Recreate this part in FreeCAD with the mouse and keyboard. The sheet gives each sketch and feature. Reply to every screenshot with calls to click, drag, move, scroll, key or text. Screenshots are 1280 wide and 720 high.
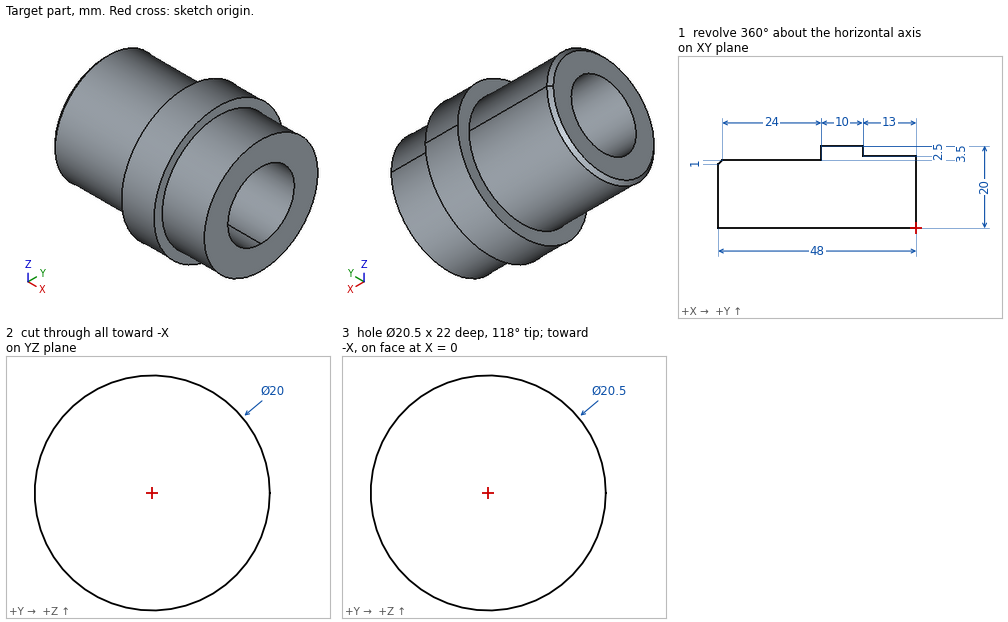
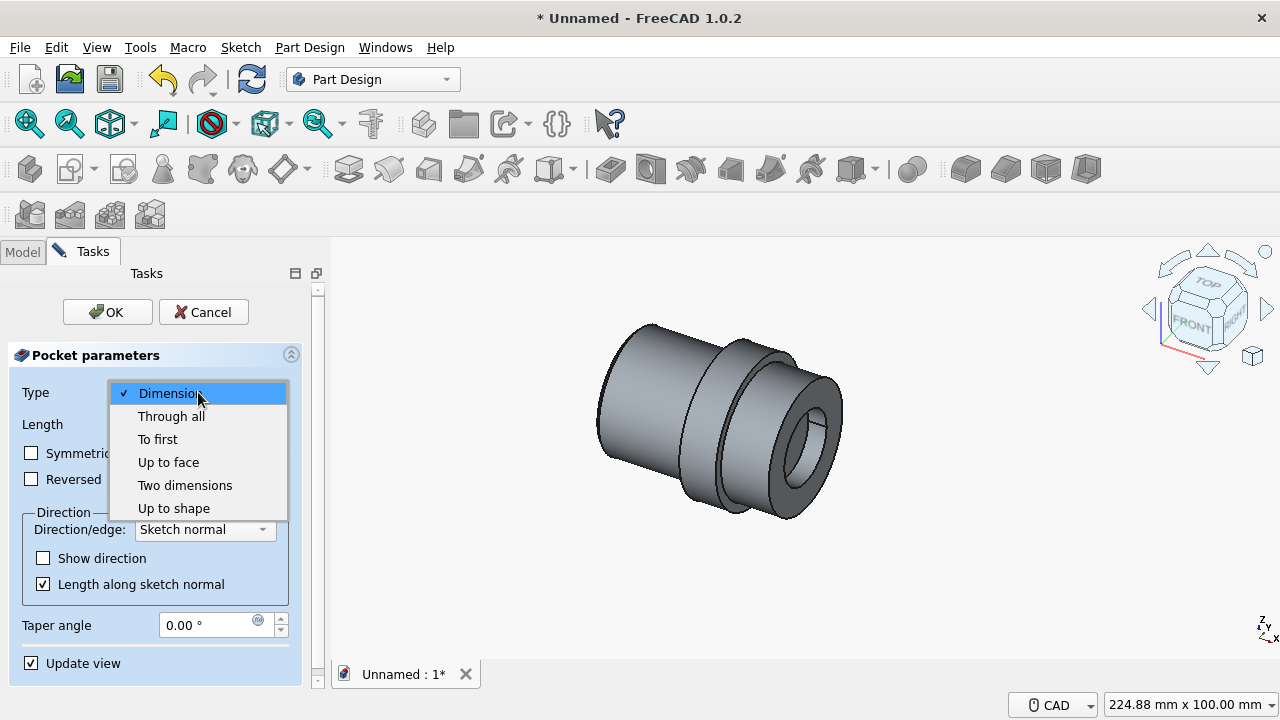
click(198, 416)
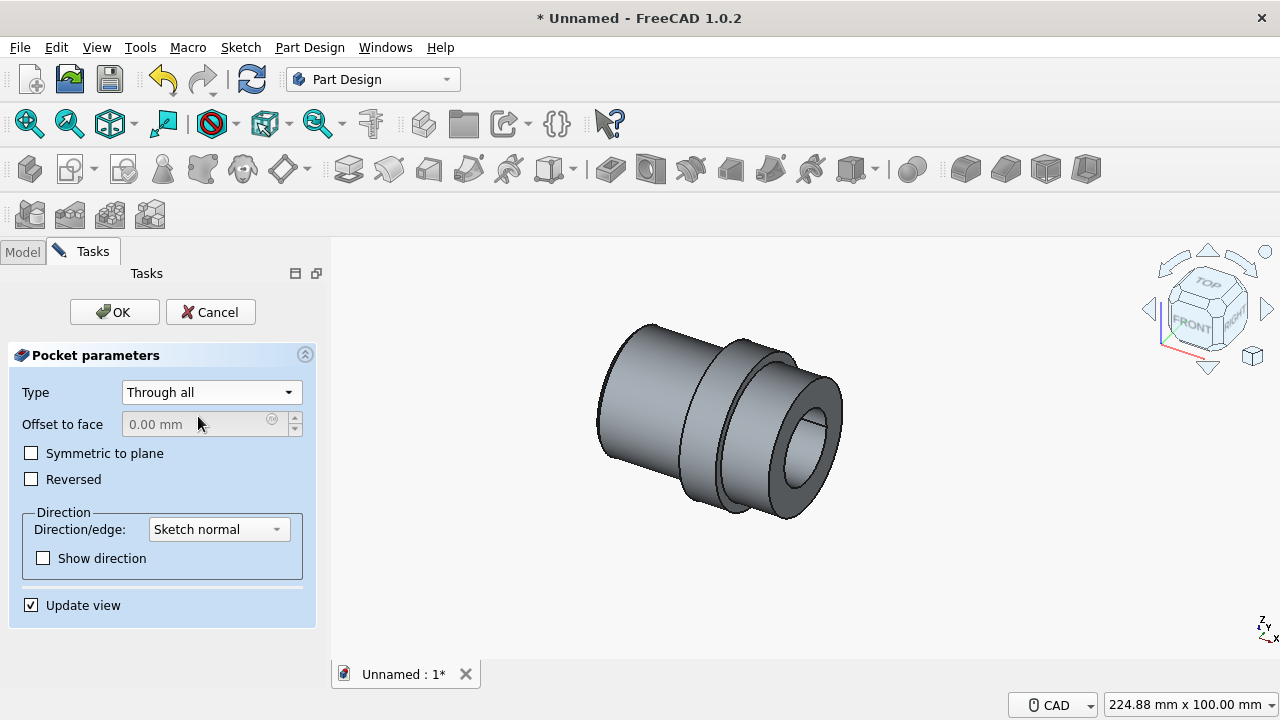
click(115, 312)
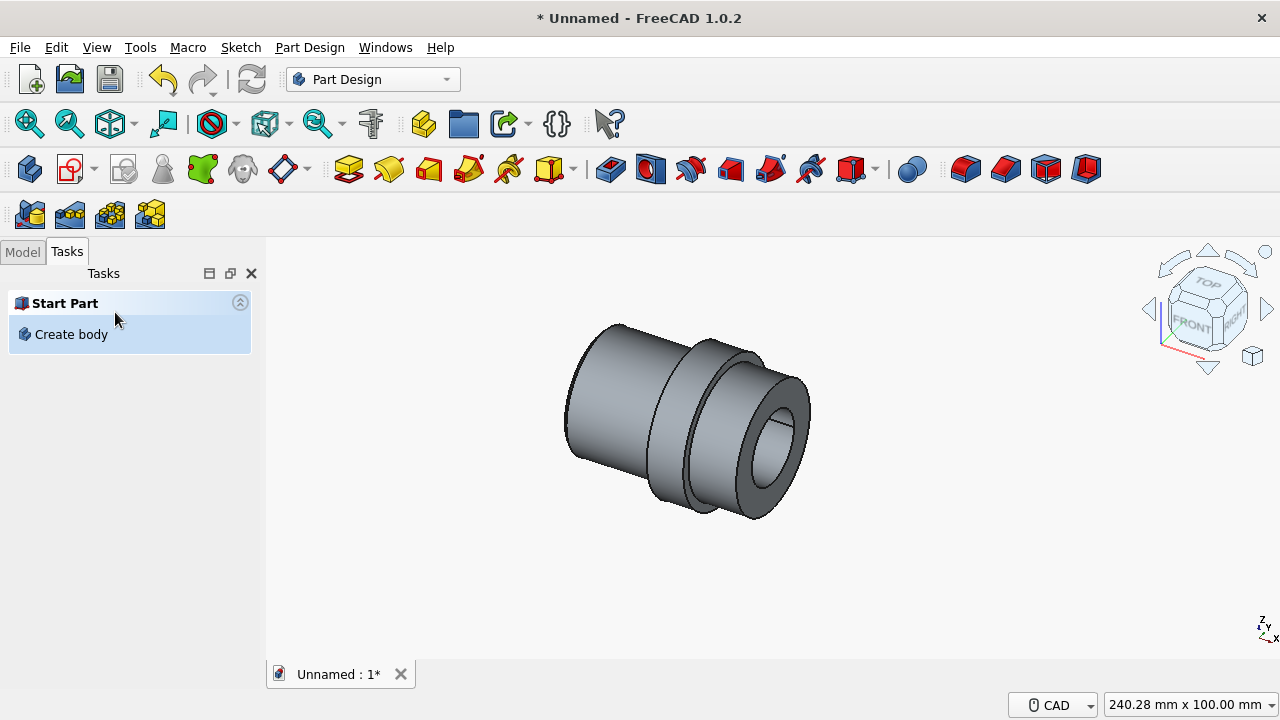
click(752, 503)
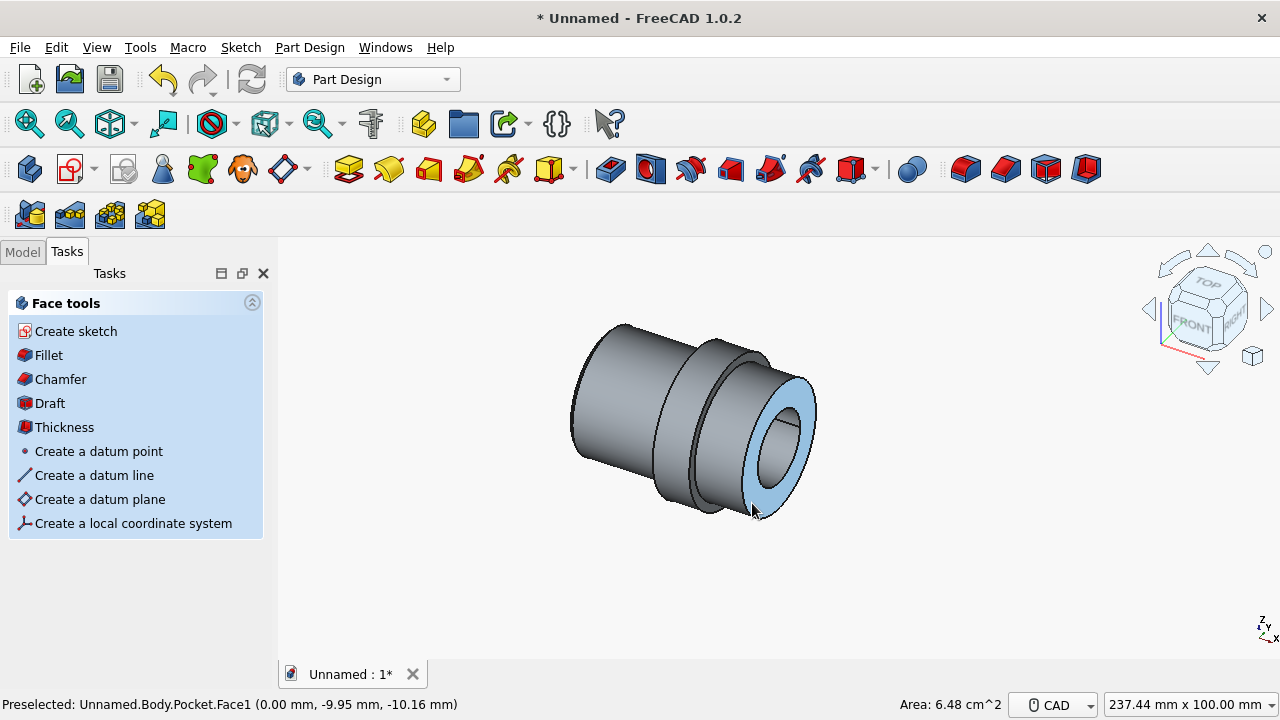
click(70, 170)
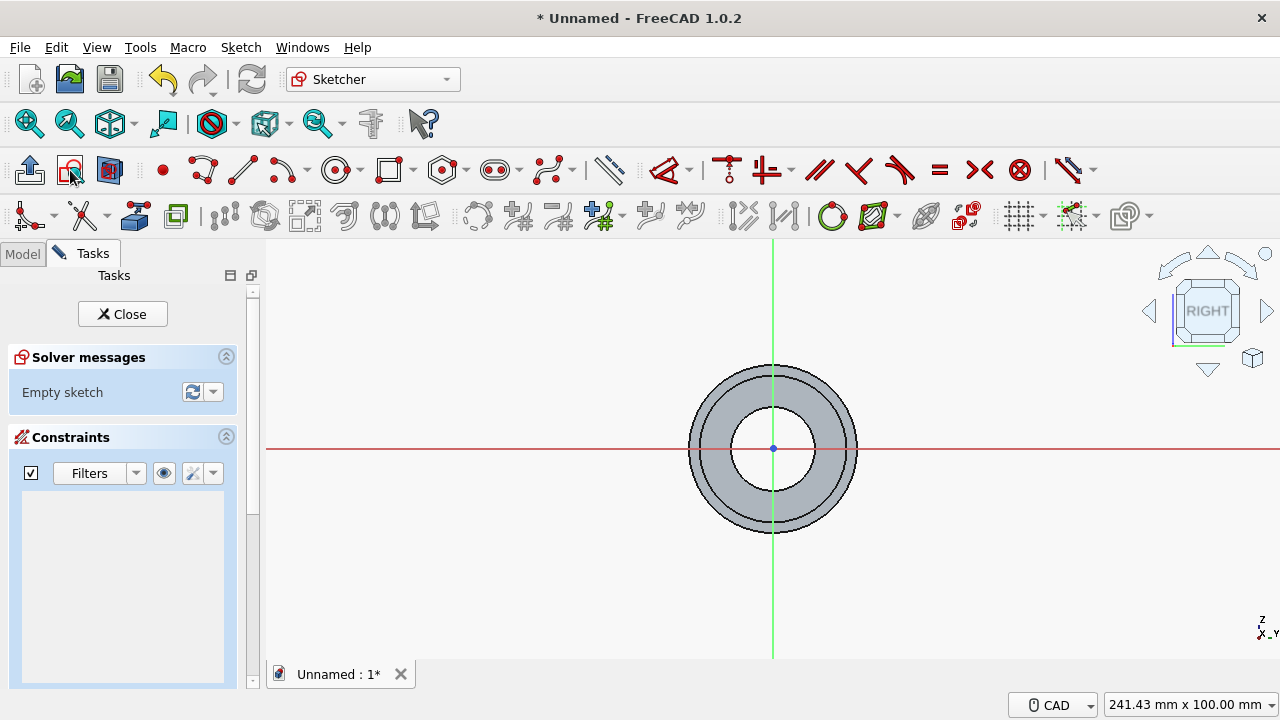
scroll(813, 449, up, 5)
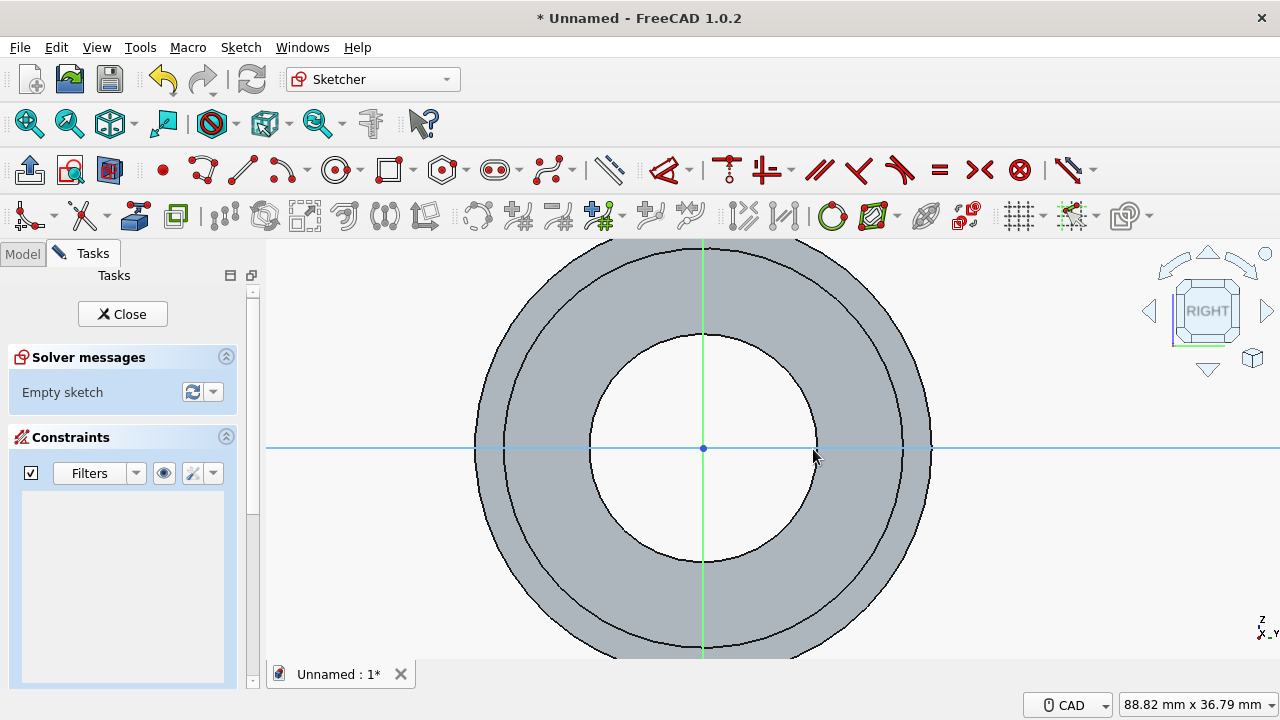
key(g)
key(c)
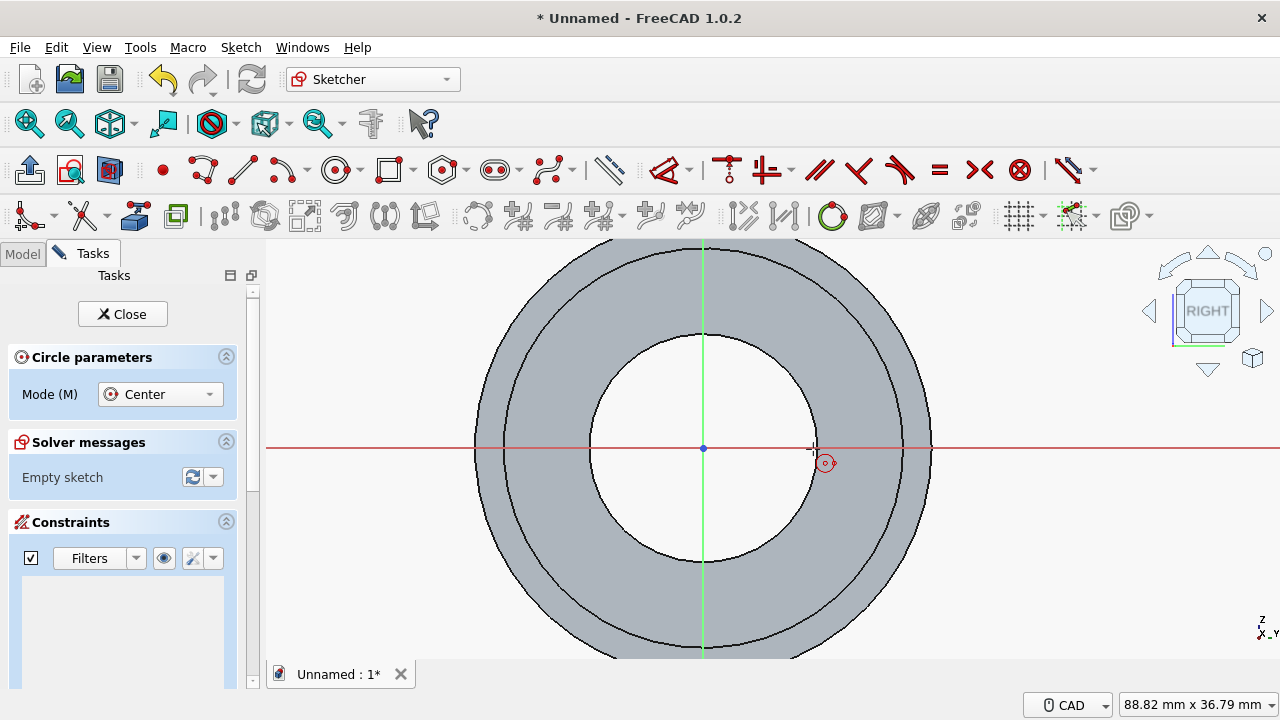
click(703, 448)
move(786, 365)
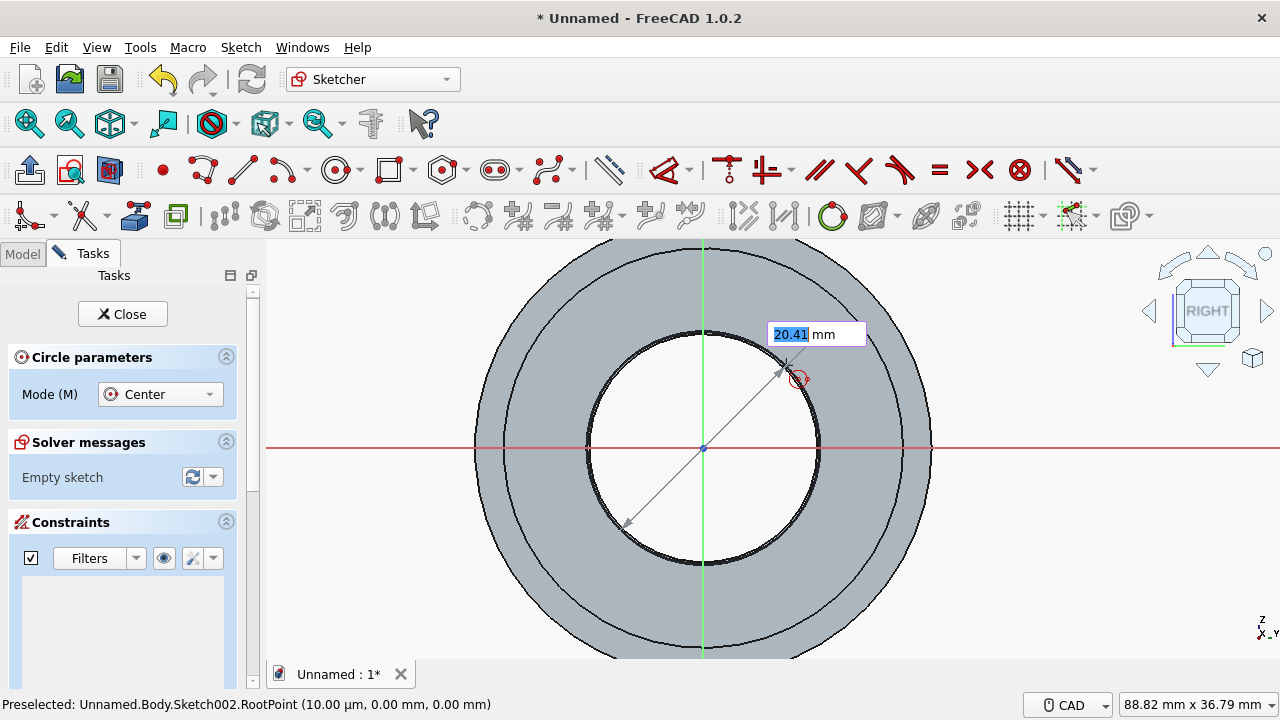
text(20.5)
key(Return)
key(Escape)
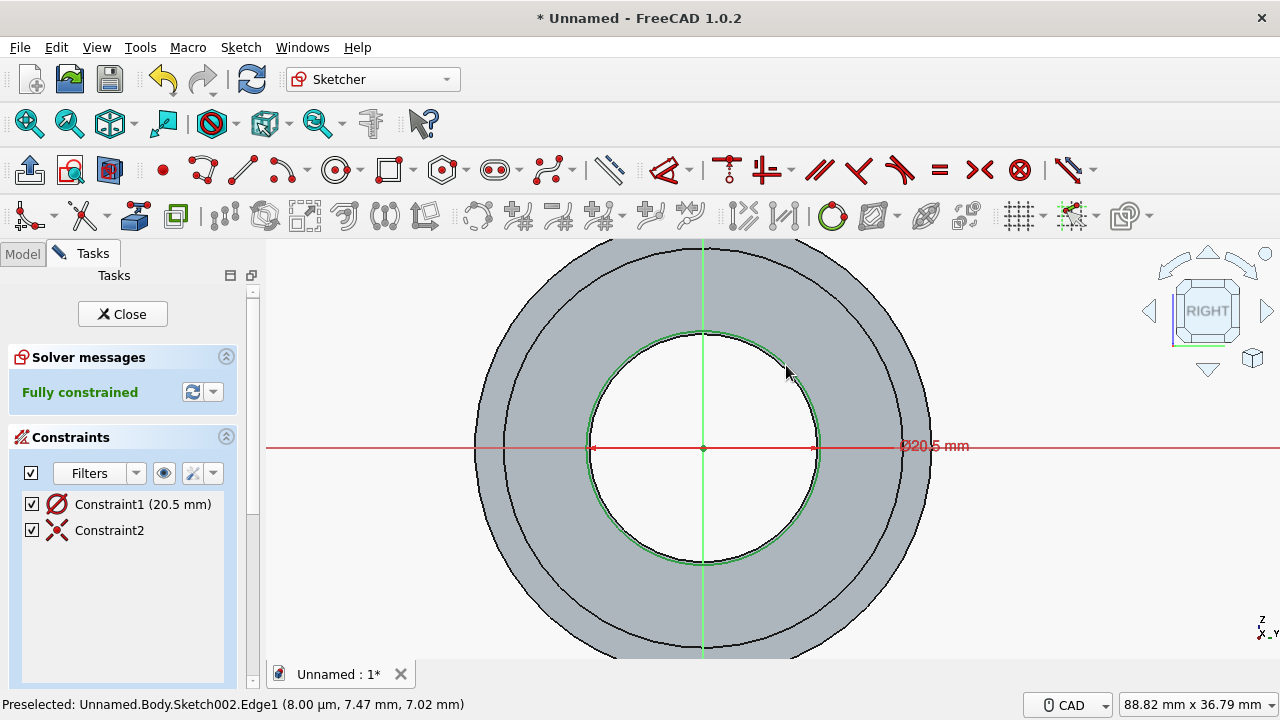
click(123, 314)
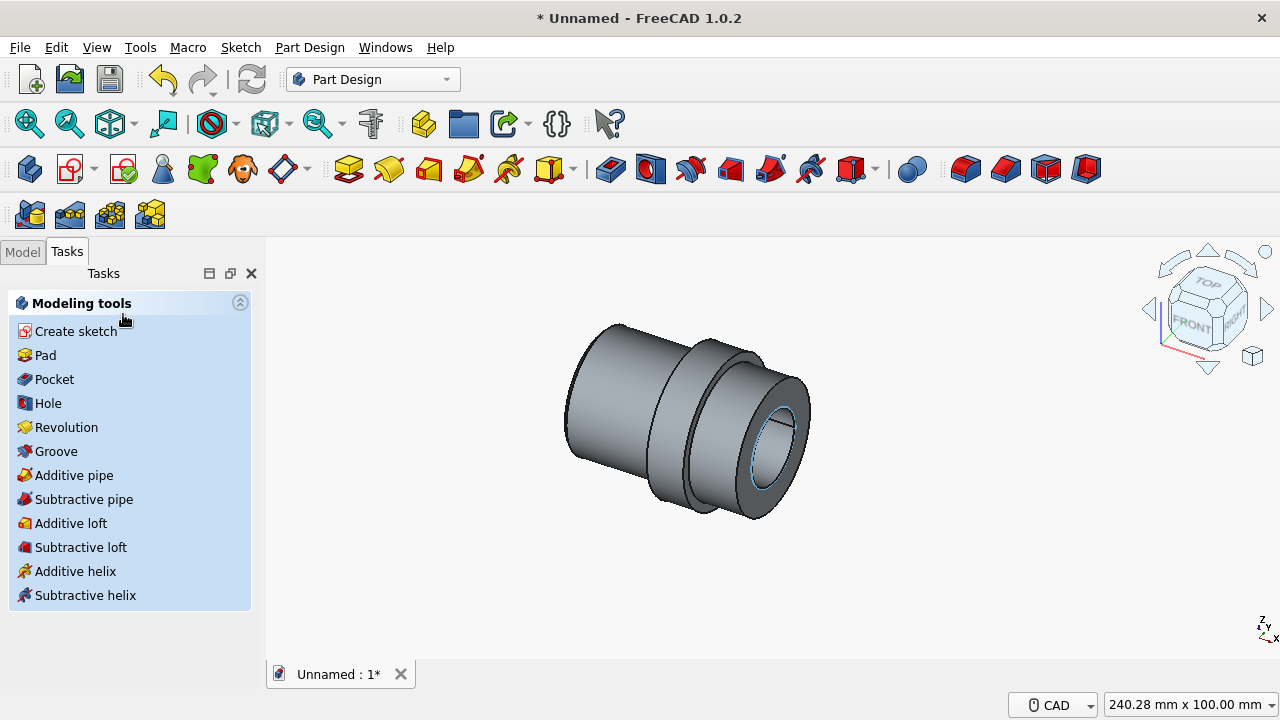
click(652, 170)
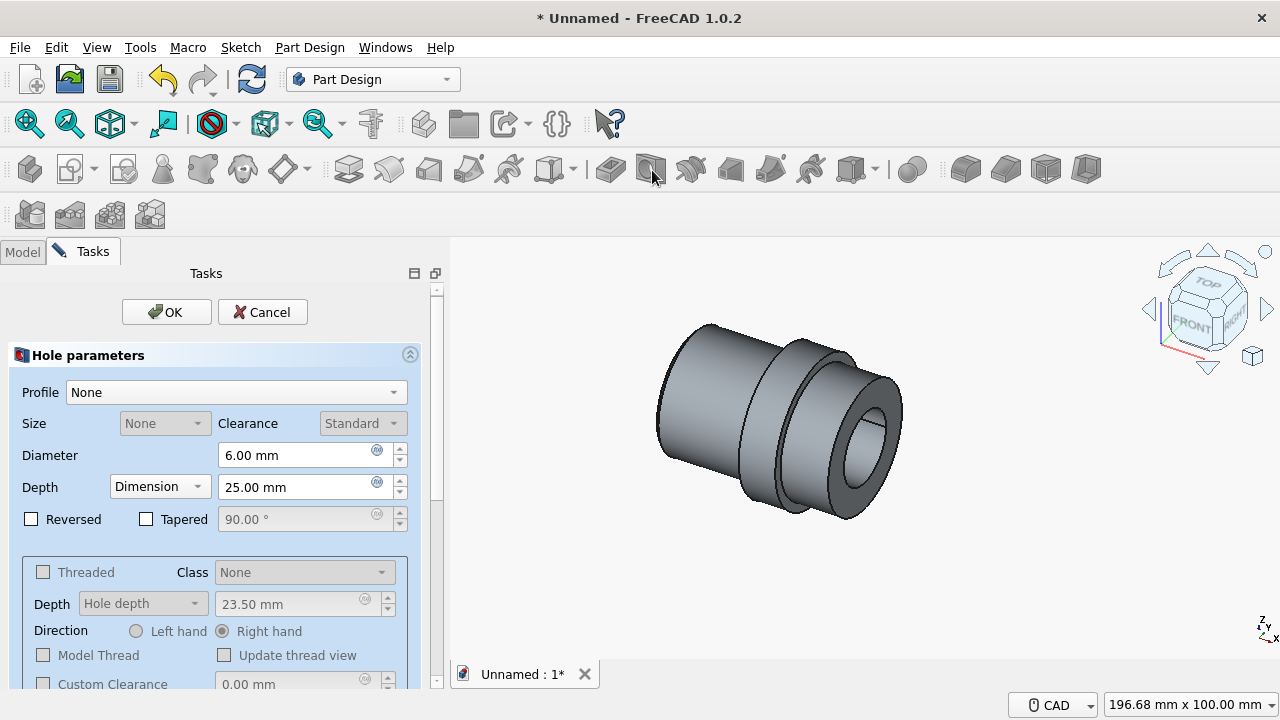
triple_click(305, 455)